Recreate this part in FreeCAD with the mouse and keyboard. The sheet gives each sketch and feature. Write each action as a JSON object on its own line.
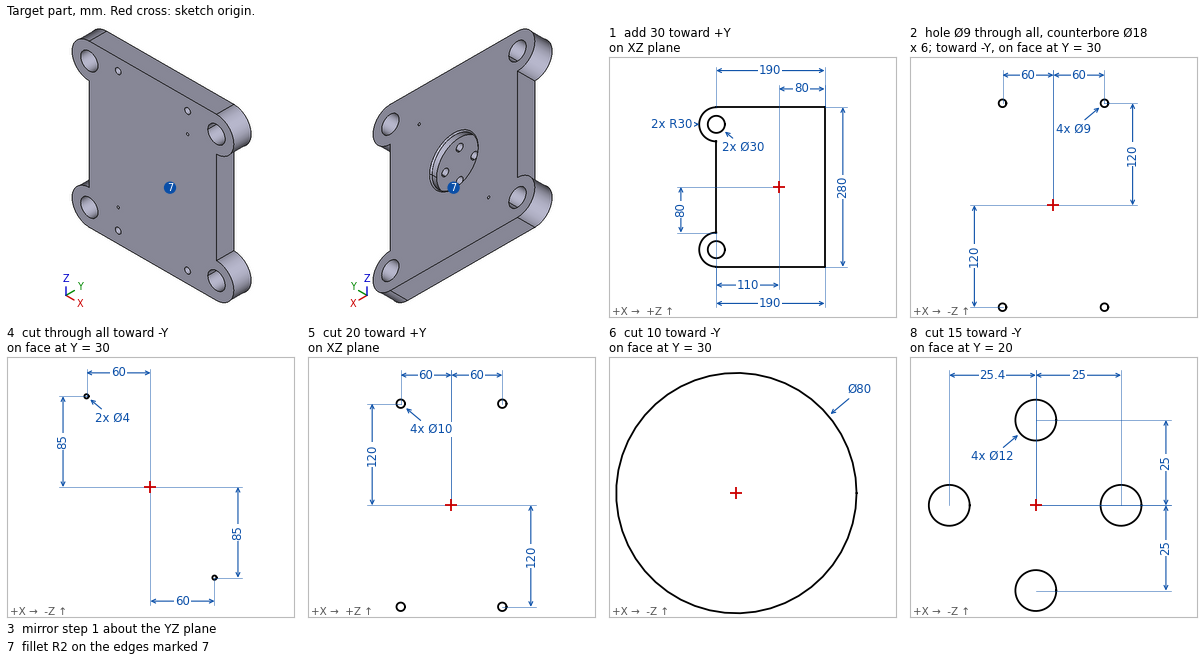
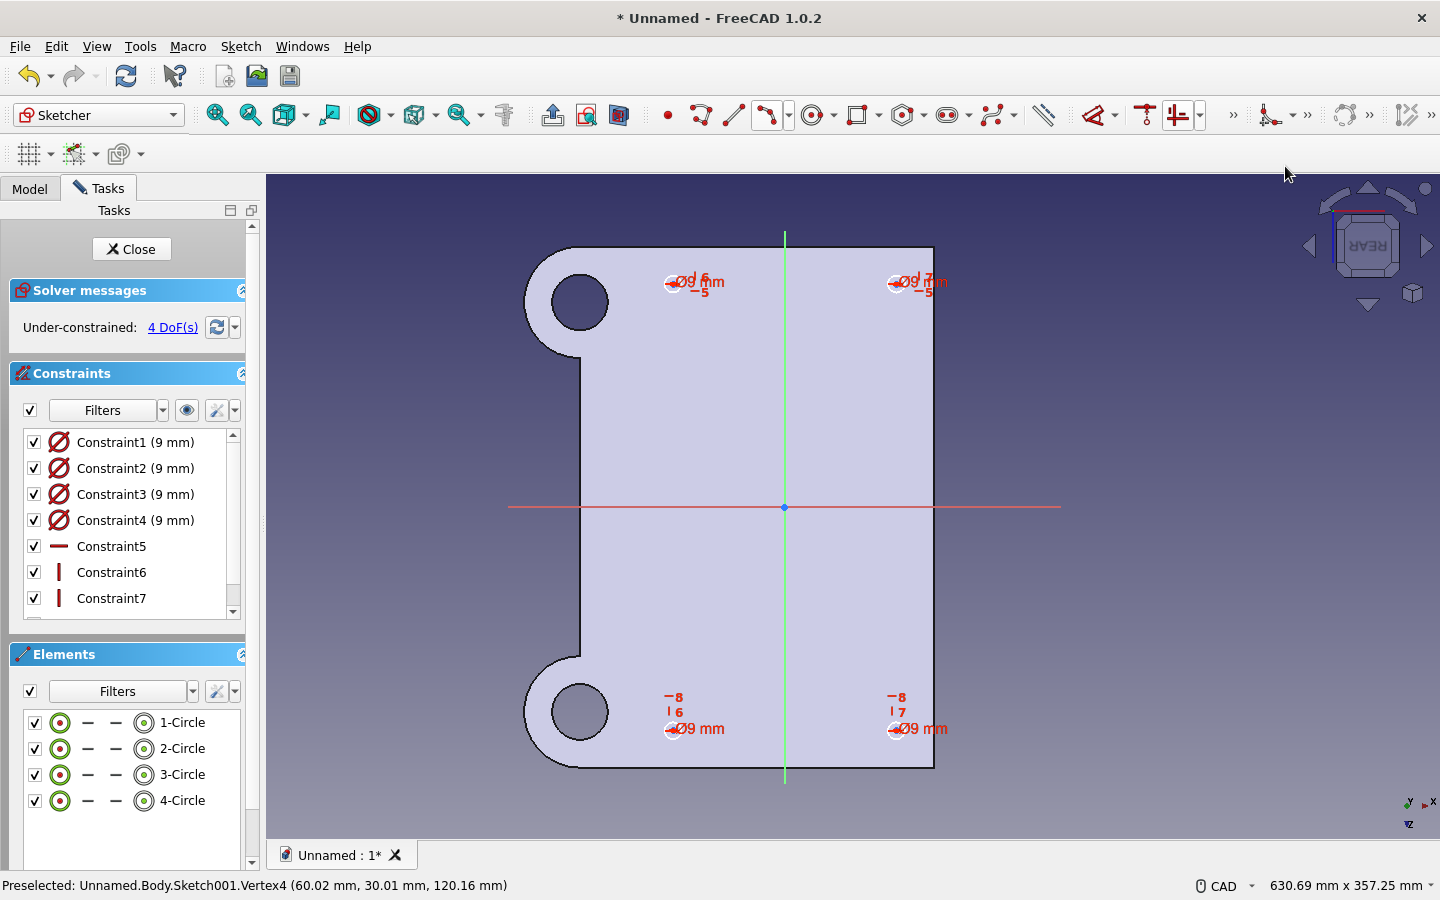
{"action": "key", "text": "d"}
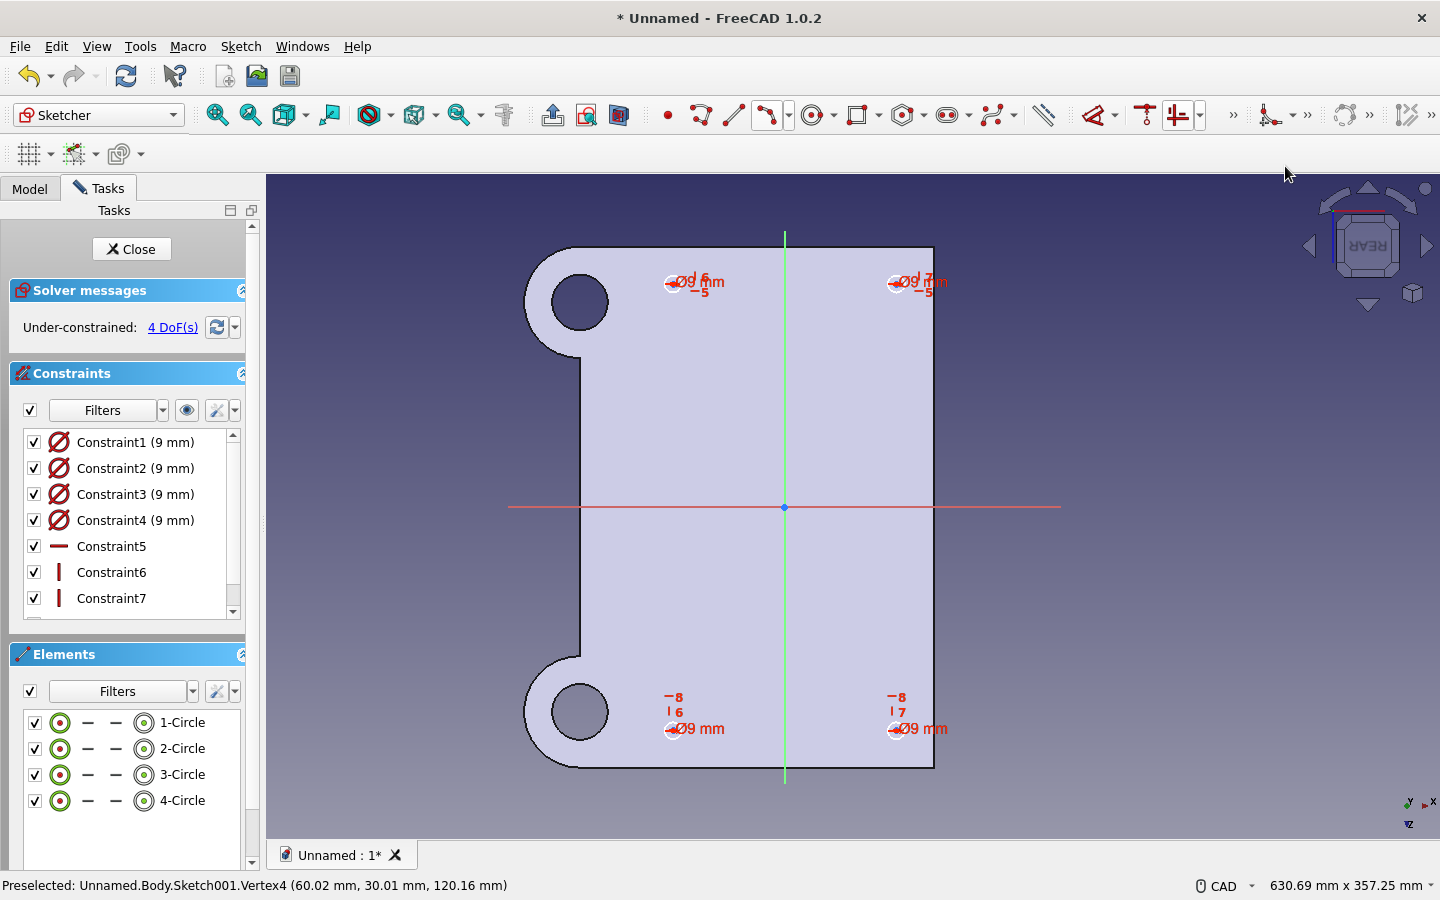
{"action": "left_click", "coordinate": [896, 284]}
{"action": "left_click", "coordinate": [841, 250]}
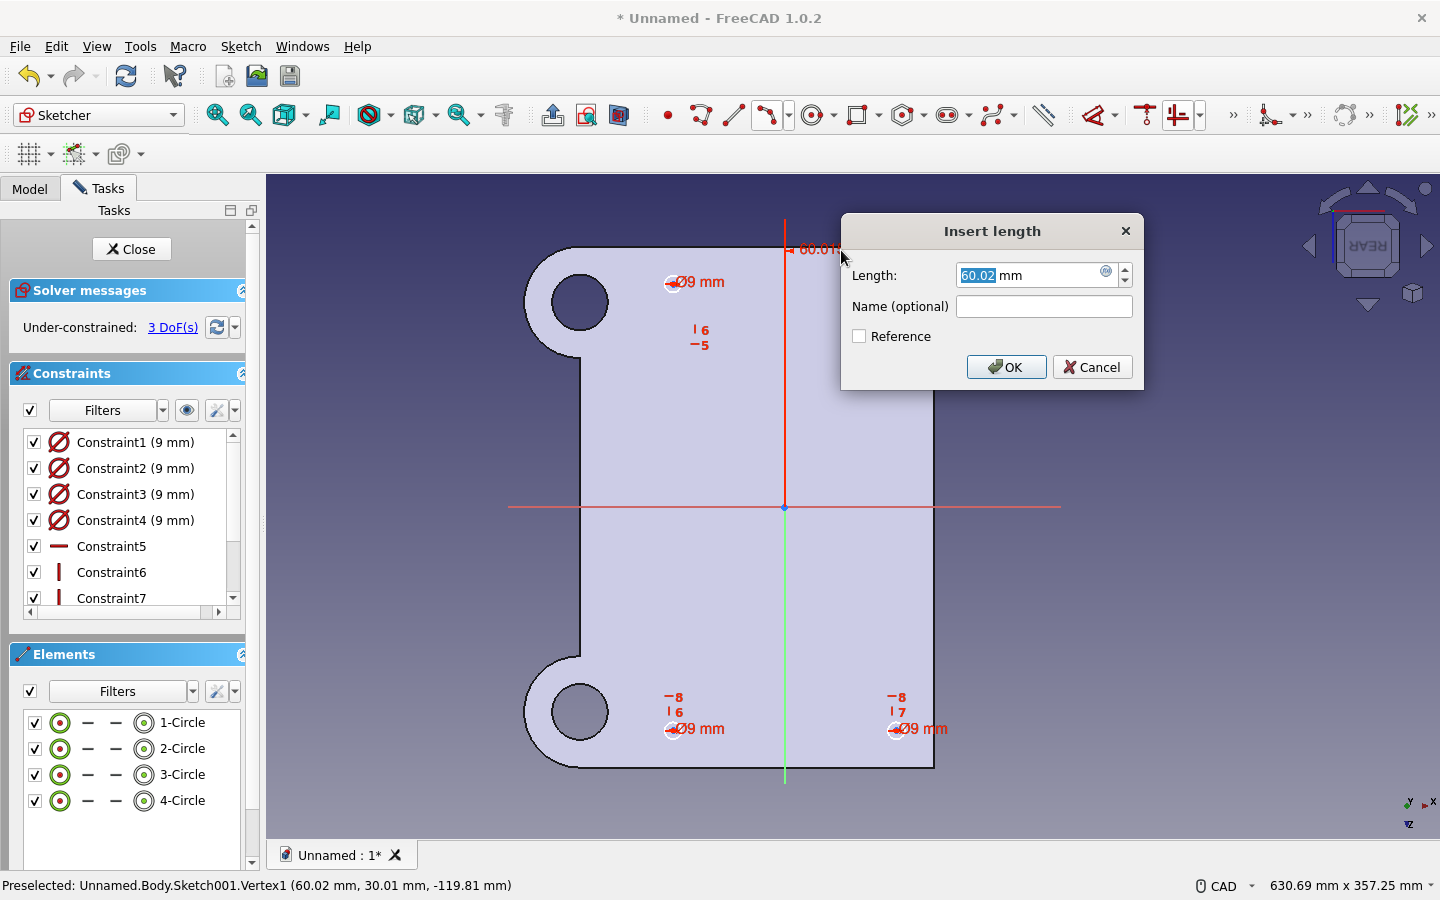
{"action": "type", "text": "60"}
{"action": "key", "text": "Return"}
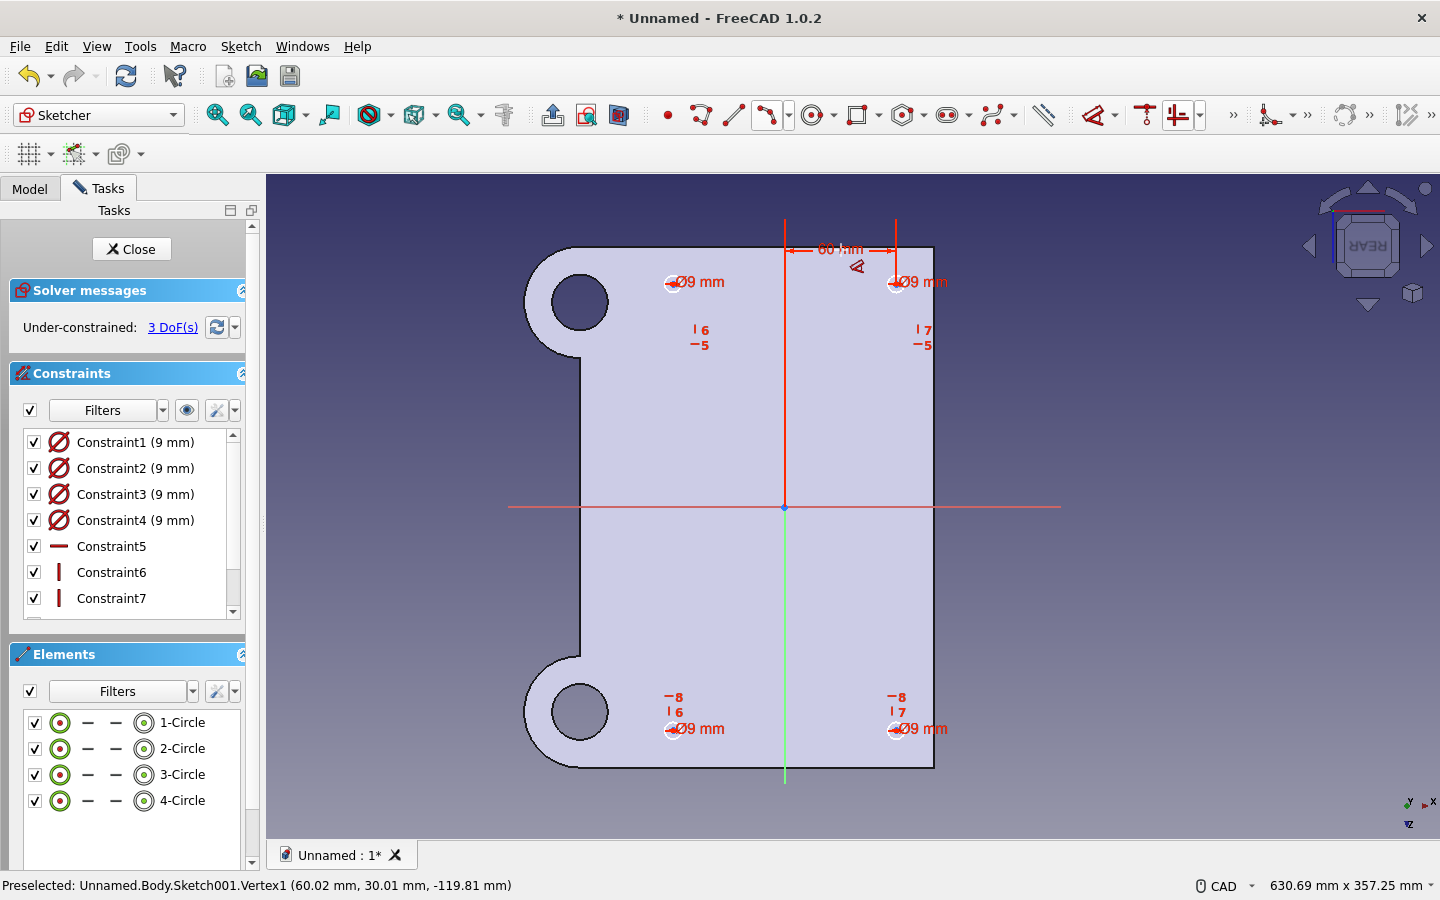
{"action": "left_click", "coordinate": [673, 284]}
{"action": "left_click", "coordinate": [729, 250]}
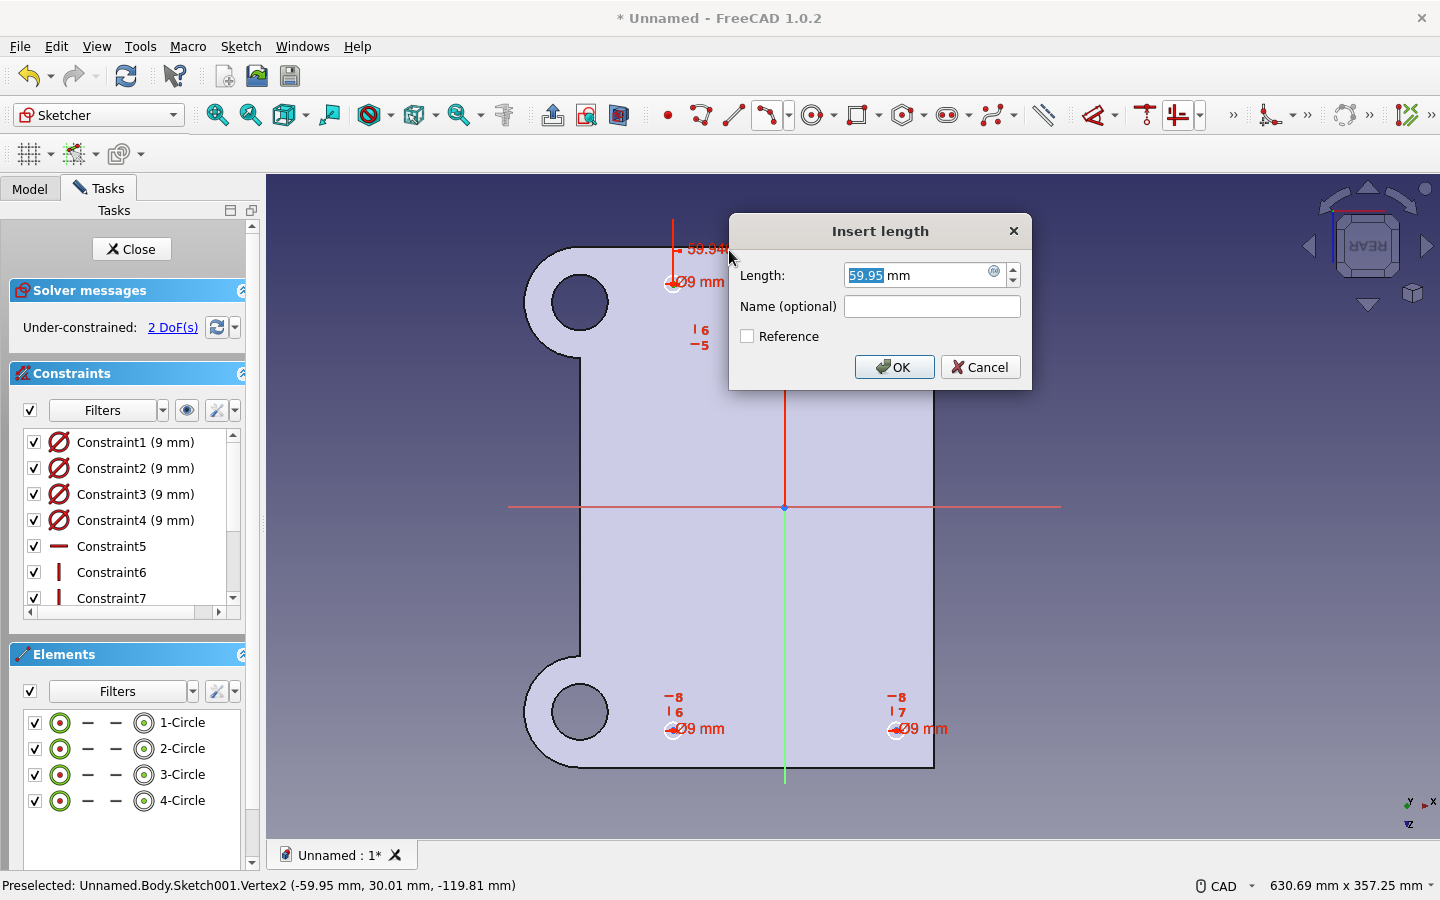
{"action": "type", "text": "60"}
{"action": "key", "text": "Return"}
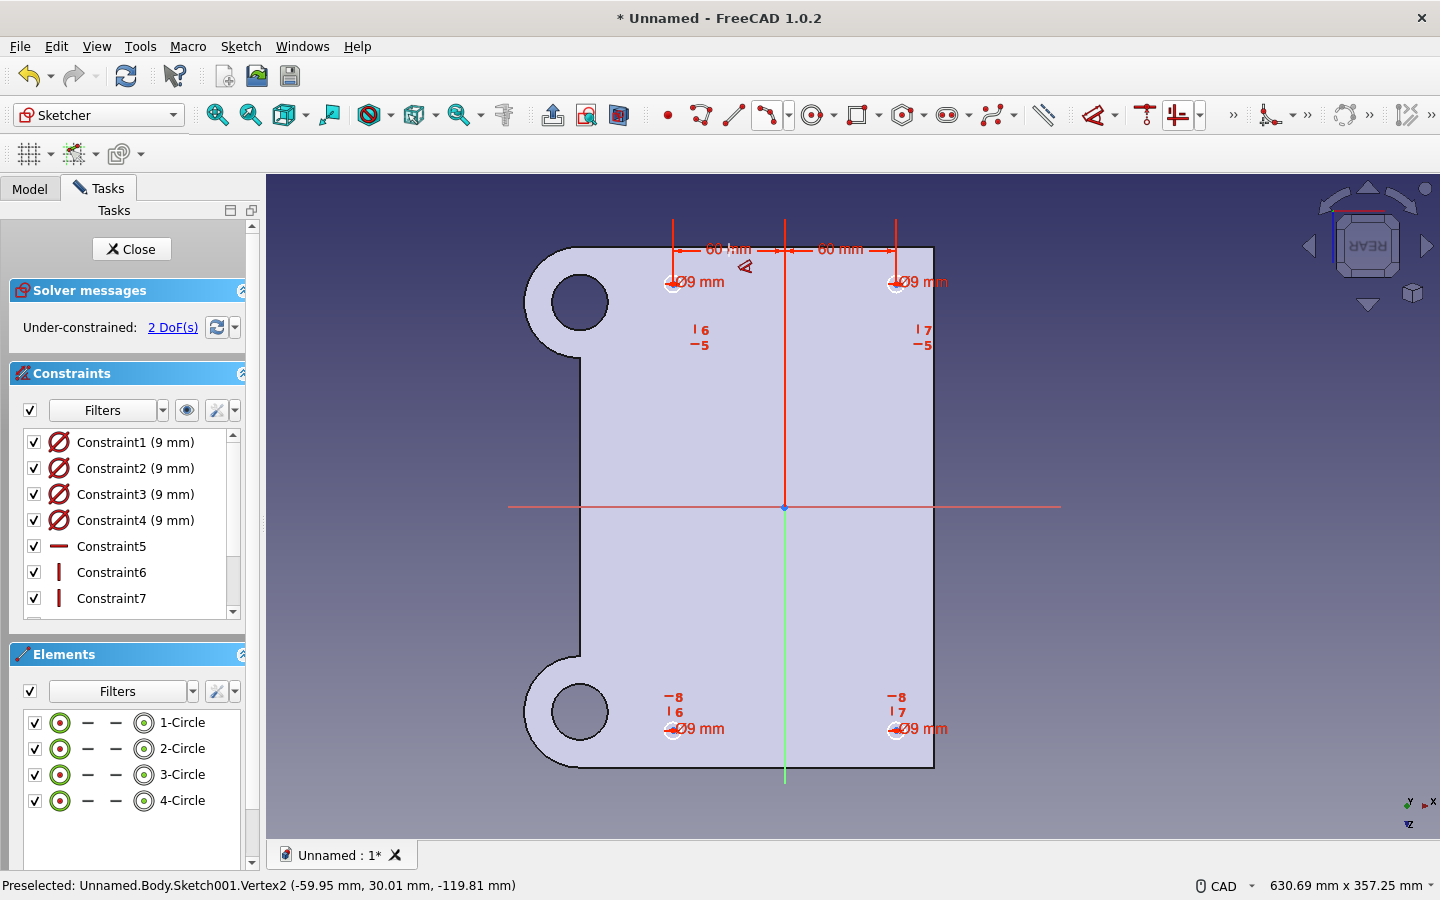
{"action": "left_click", "coordinate": [896, 284]}
{"action": "left_click", "coordinate": [930, 396]}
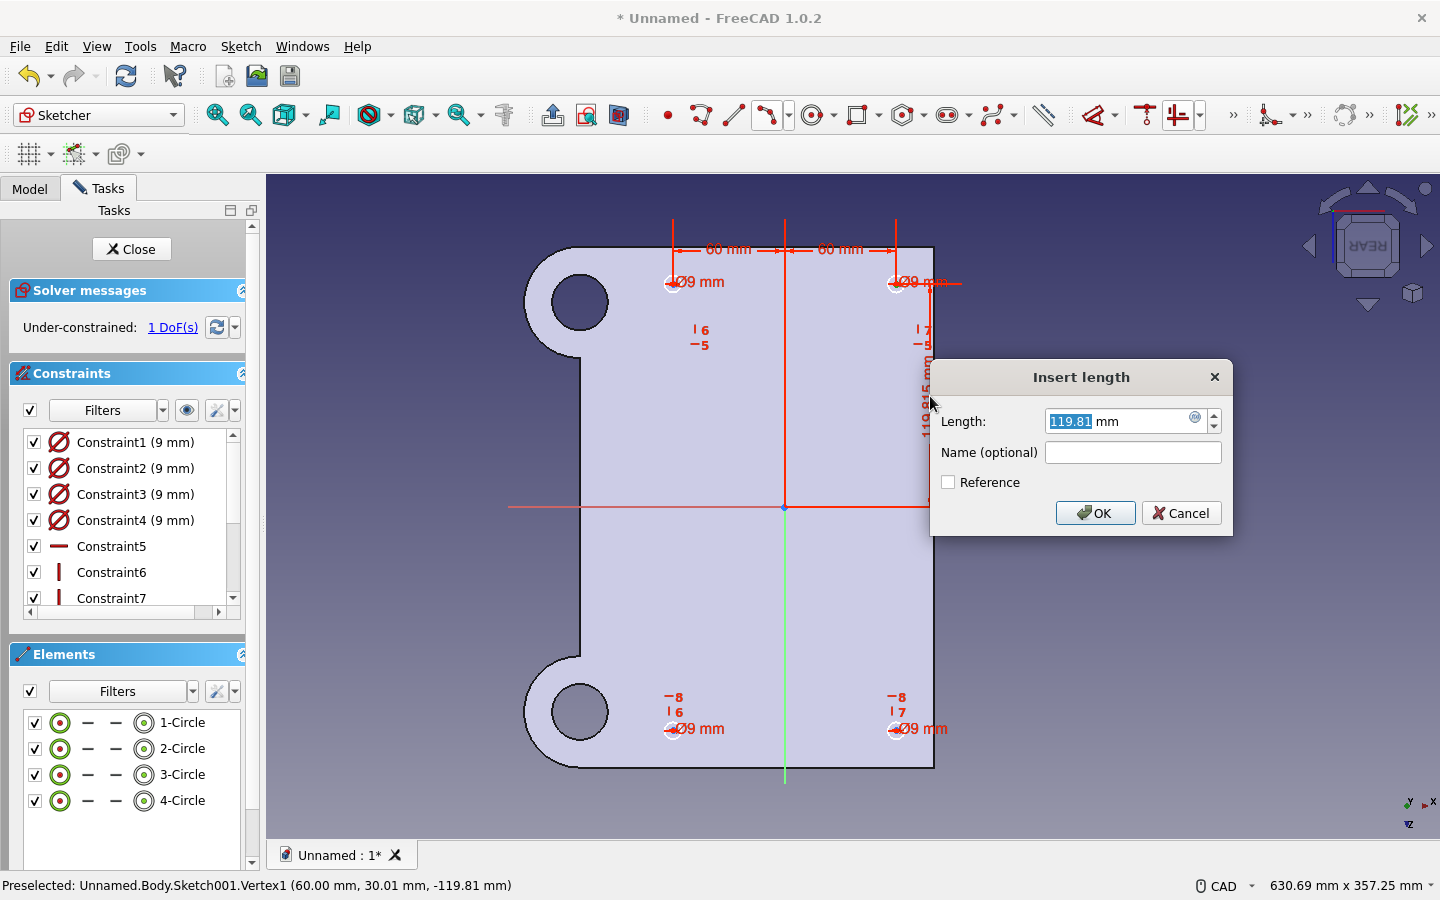
{"action": "type", "text": "120"}
{"action": "key", "text": "Return"}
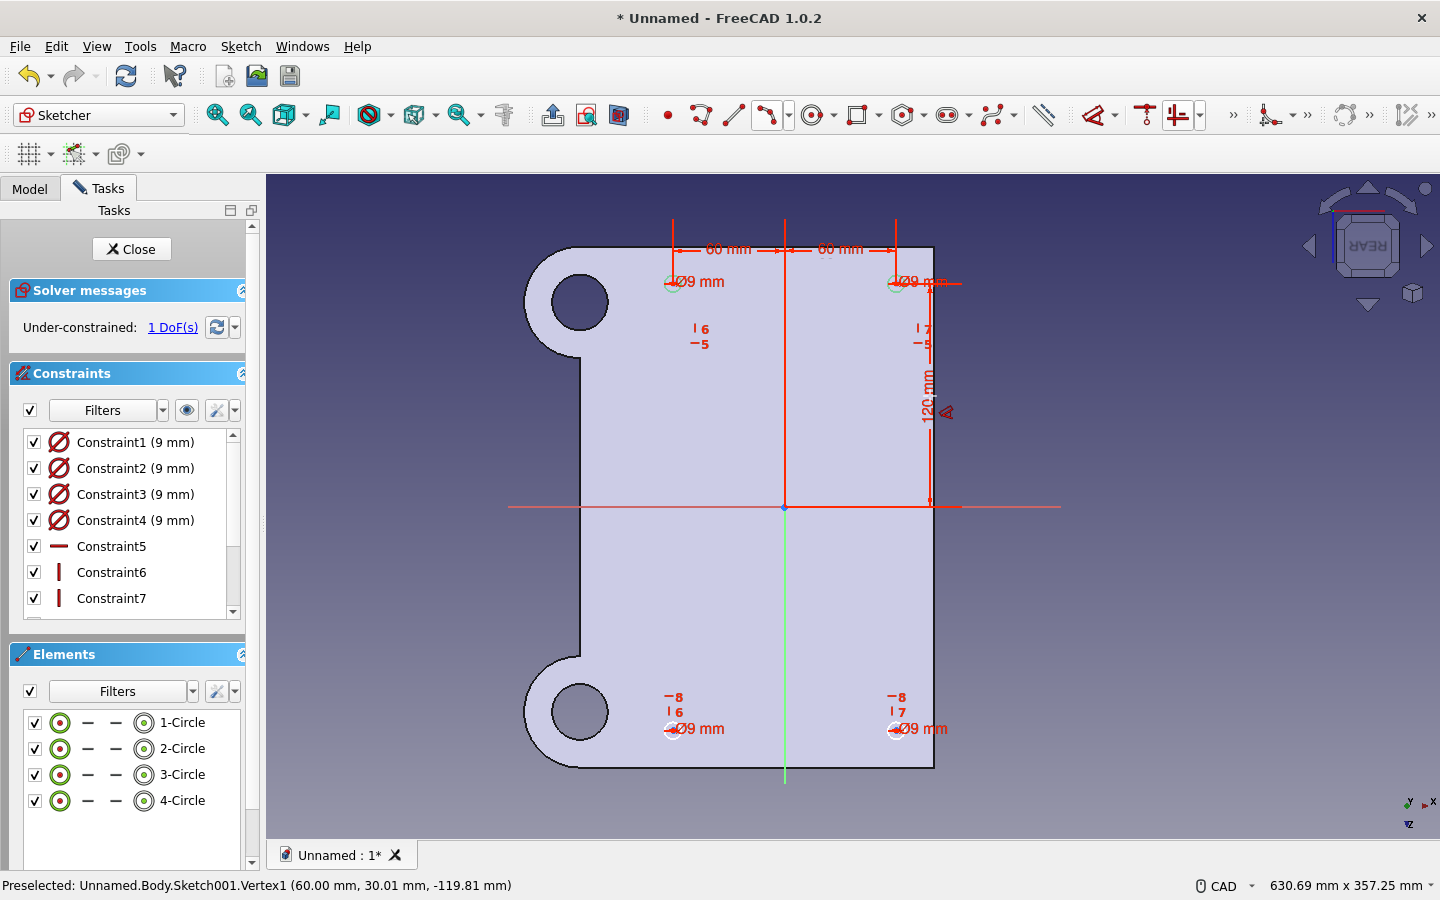
{"action": "left_click", "coordinate": [673, 731]}
{"action": "left_click", "coordinate": [639, 619]}